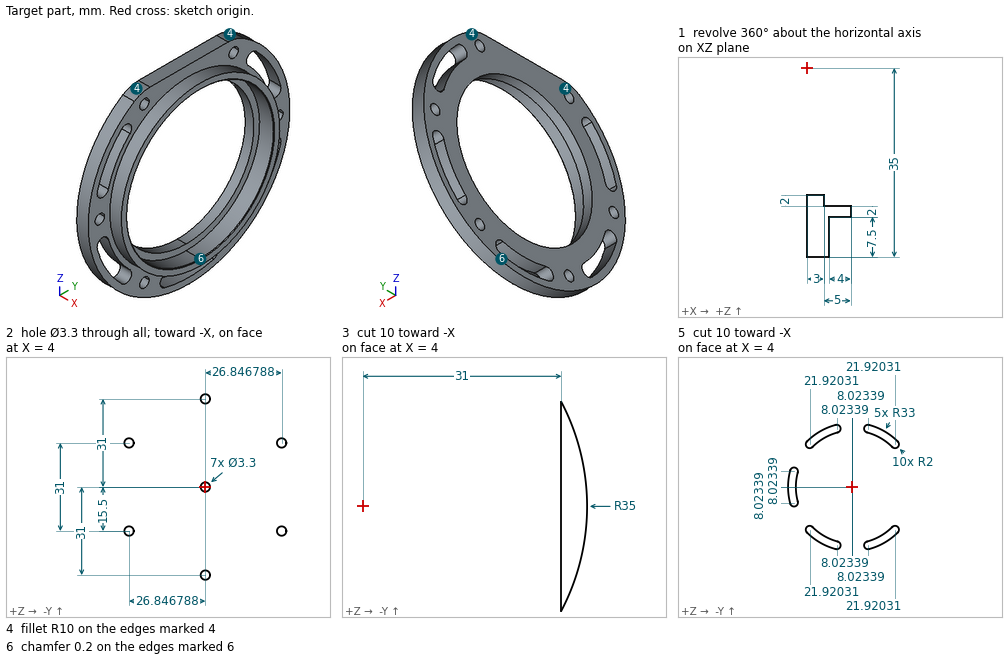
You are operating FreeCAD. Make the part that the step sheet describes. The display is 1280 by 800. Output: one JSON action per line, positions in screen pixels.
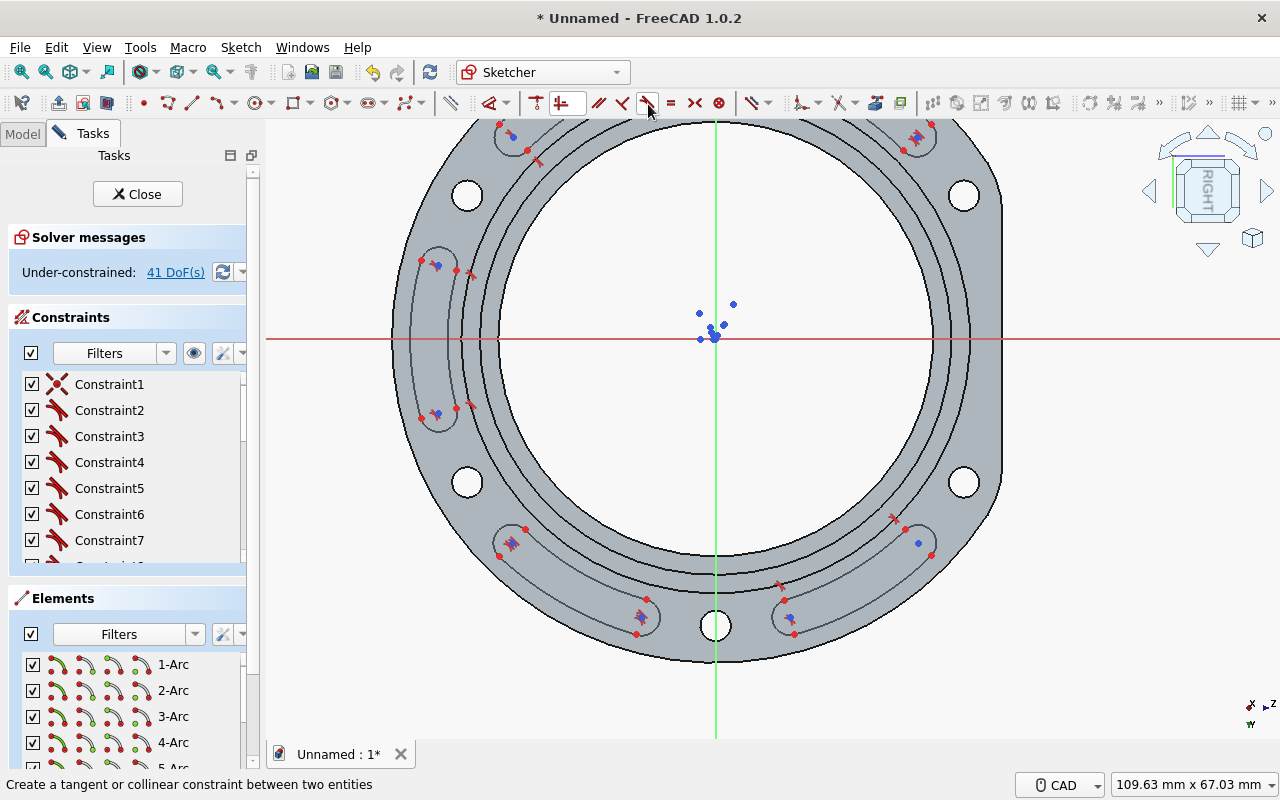
{"action": "left_click", "coordinate": [840, 618]}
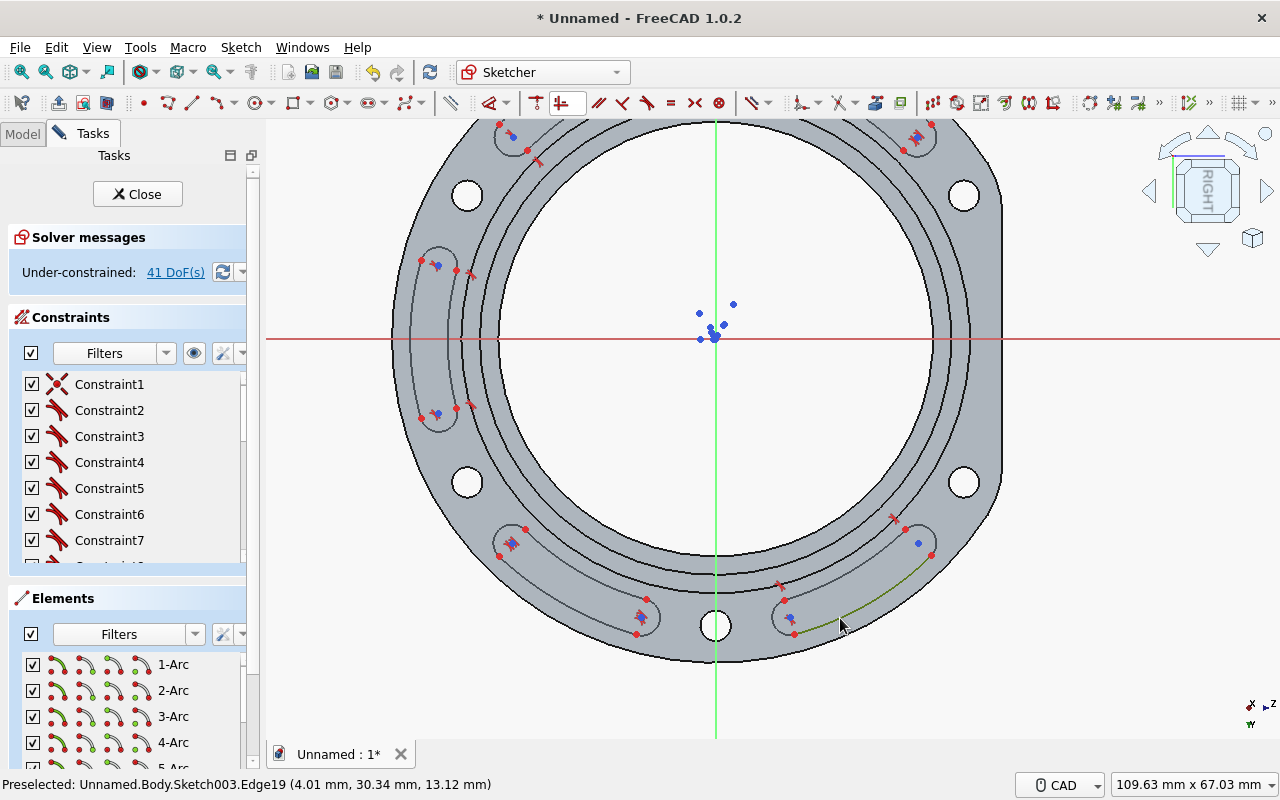
{"action": "left_click", "coordinate": [936, 540]}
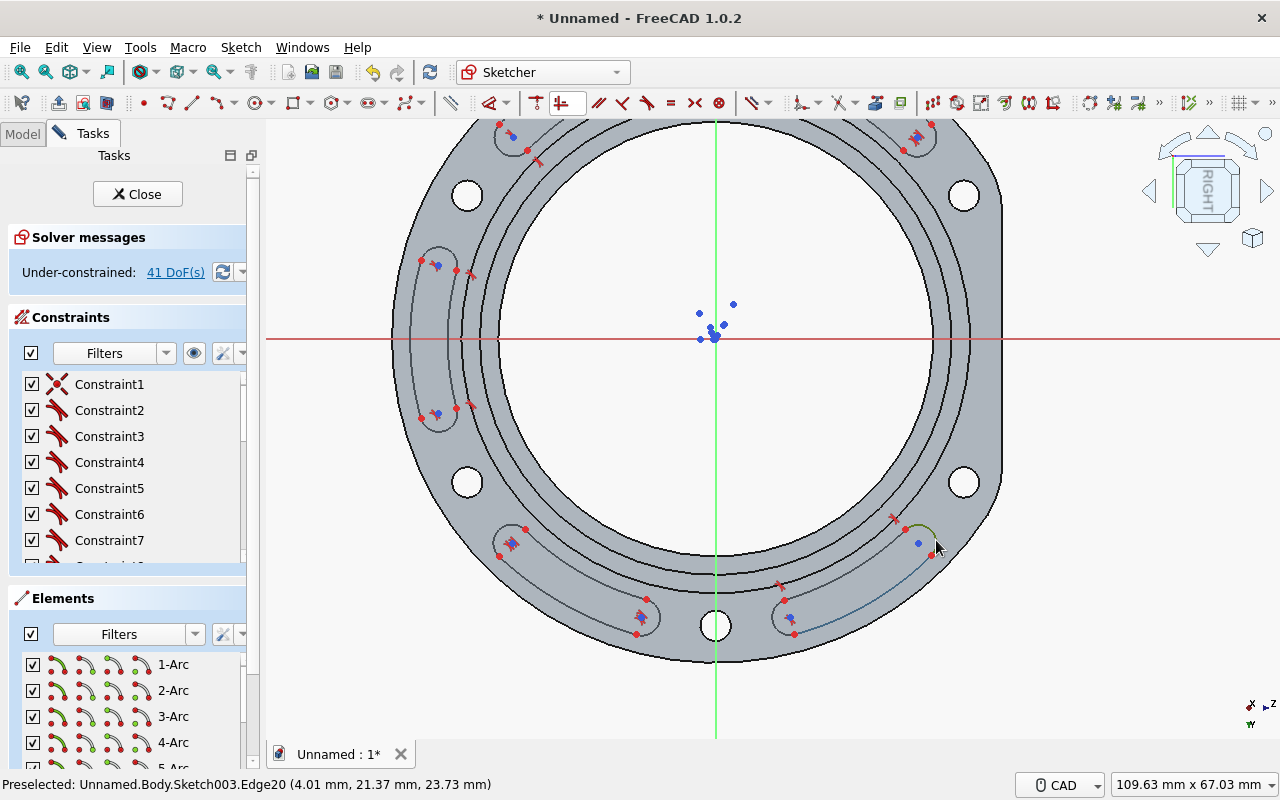
{"action": "left_click", "coordinate": [648, 104]}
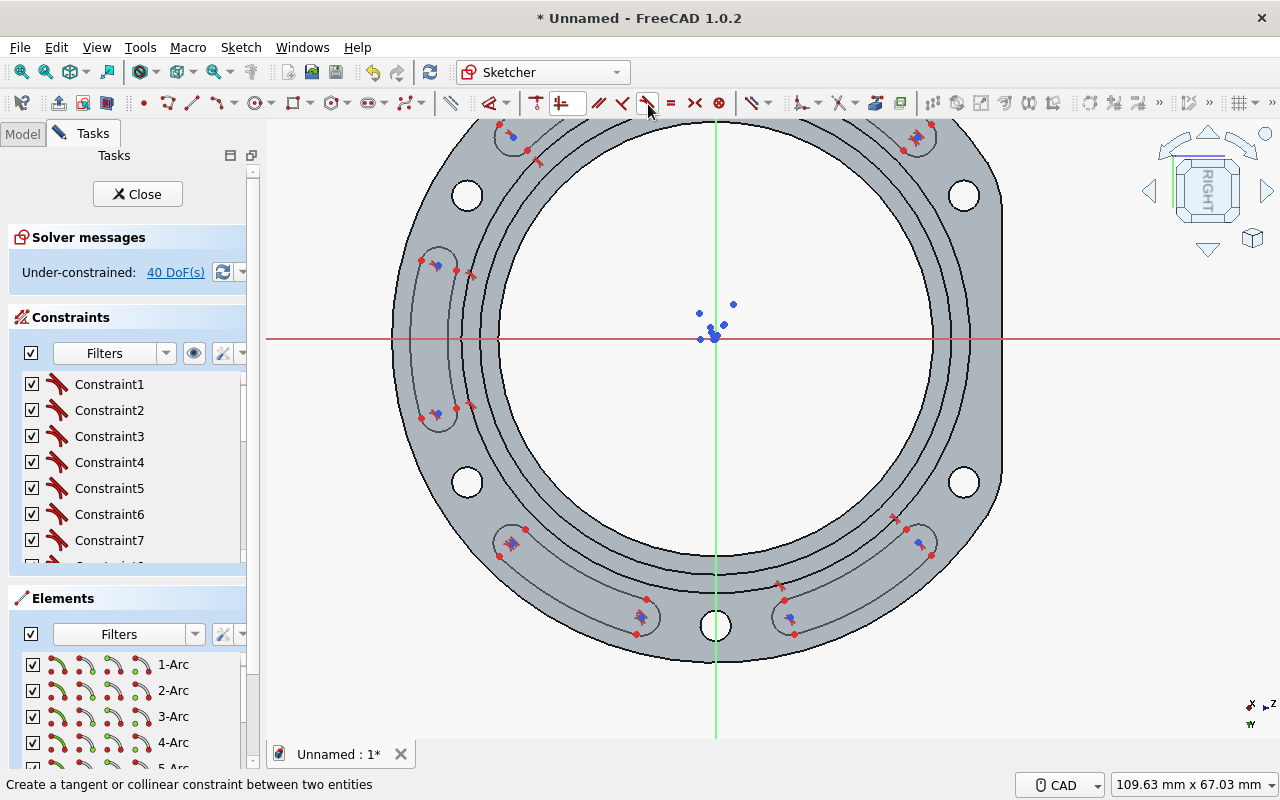
{"action": "left_click", "coordinate": [536, 587]}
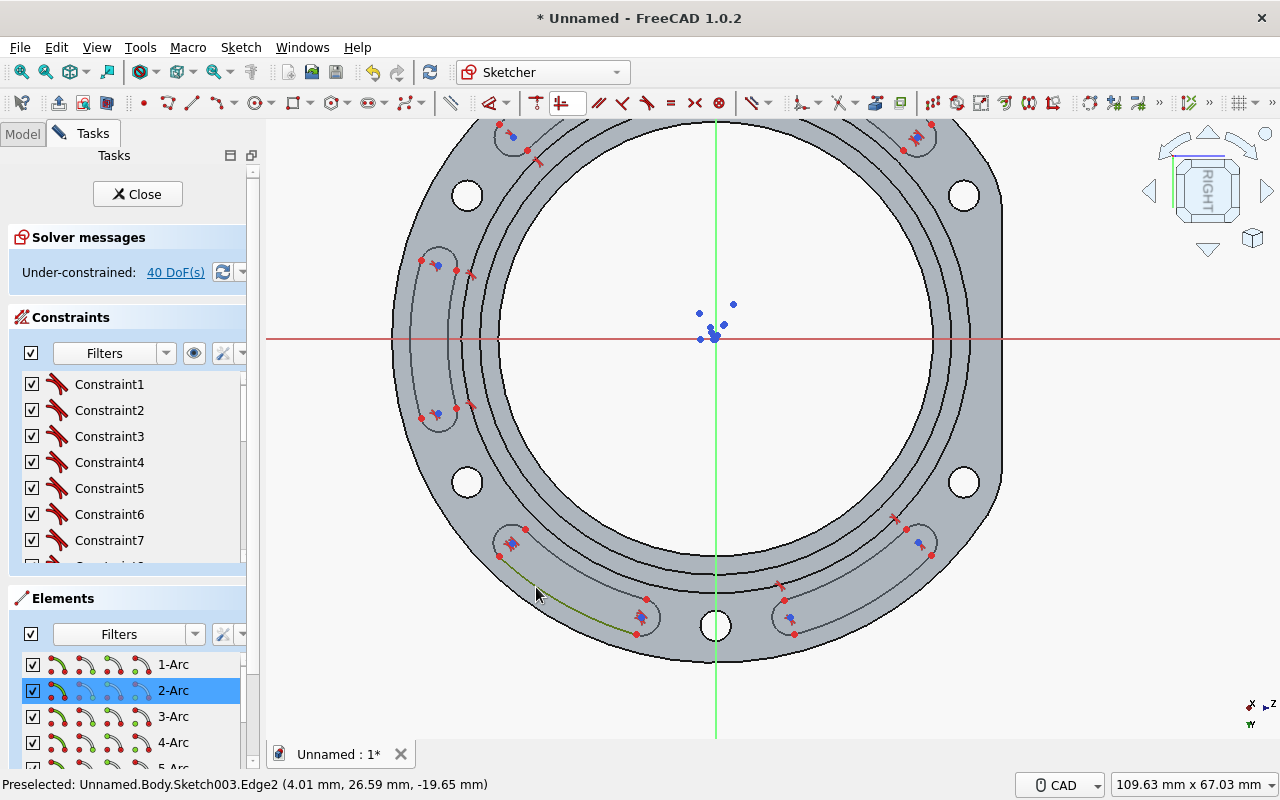
{"action": "left_click", "coordinate": [557, 557]}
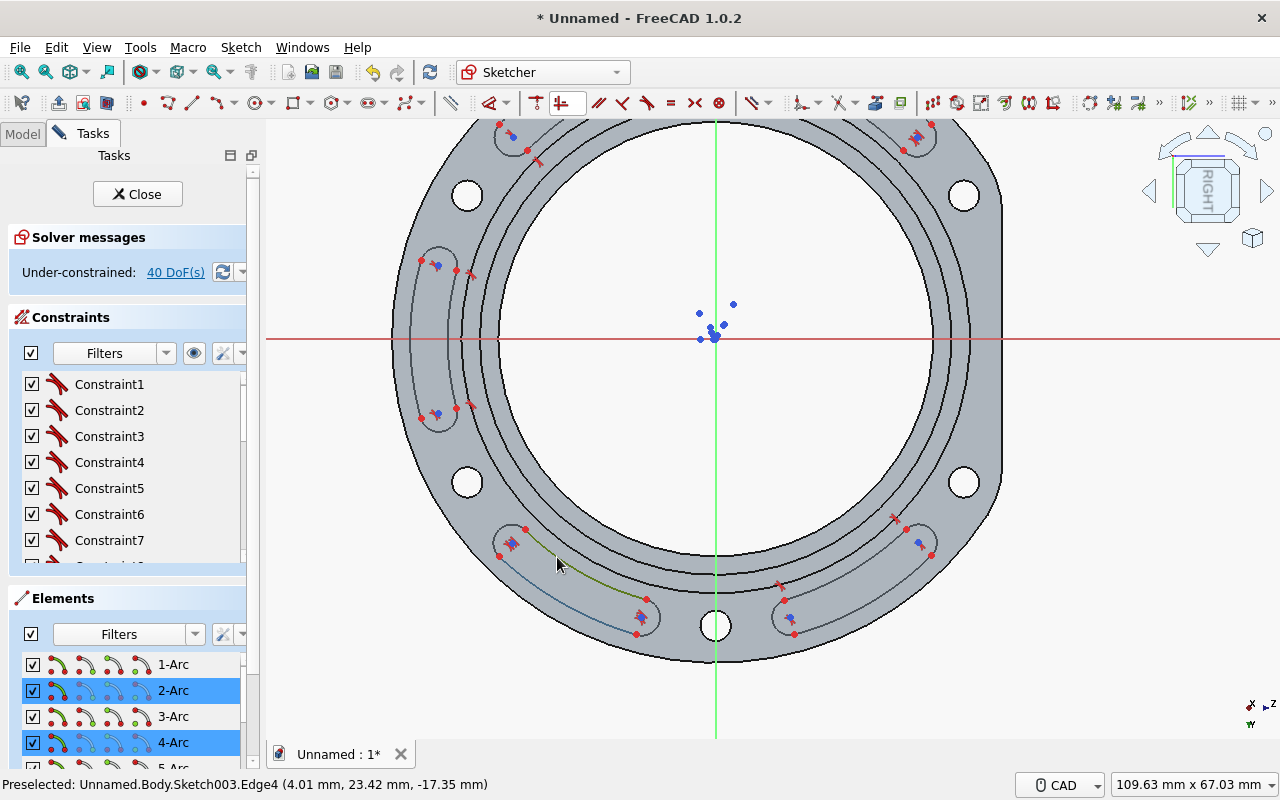
{"action": "left_click", "coordinate": [536, 104]}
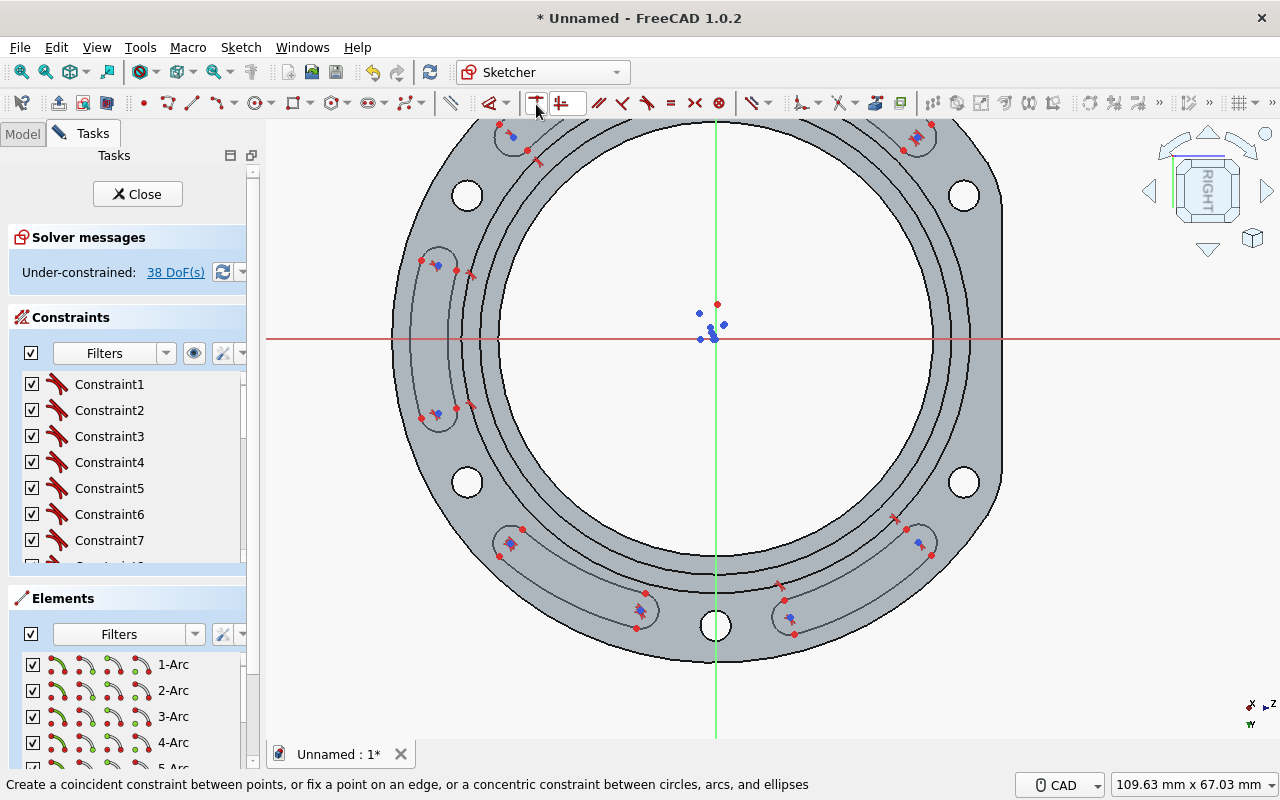
{"action": "left_click", "coordinate": [537, 585]}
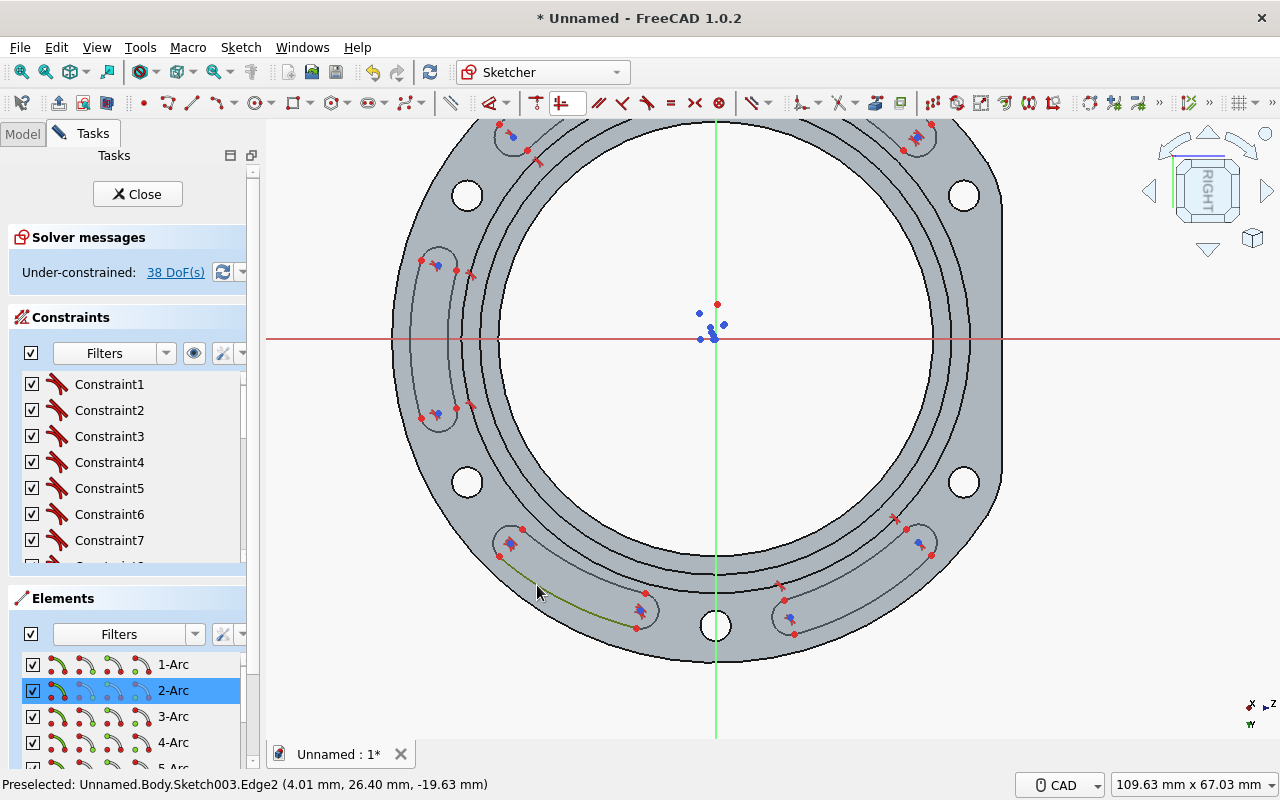
{"action": "left_click", "coordinate": [449, 312]}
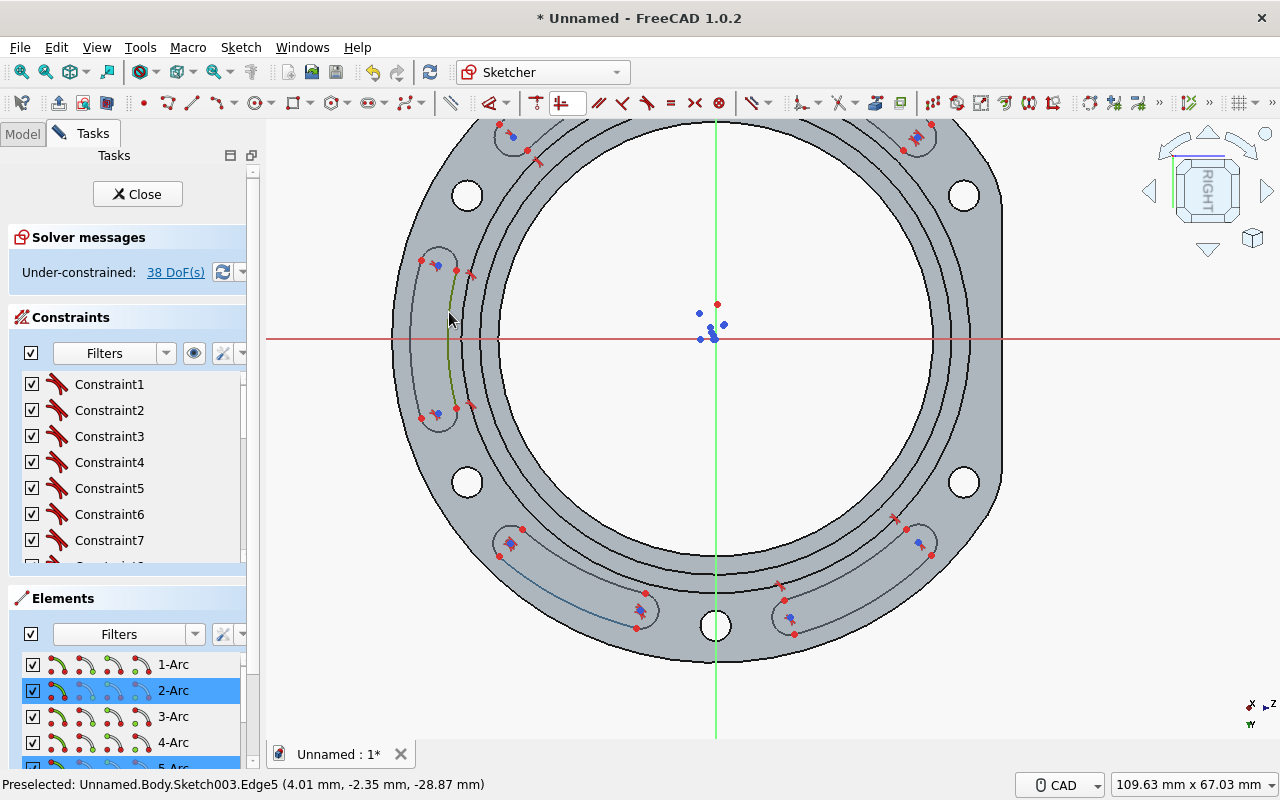
{"action": "left_click", "coordinate": [536, 104]}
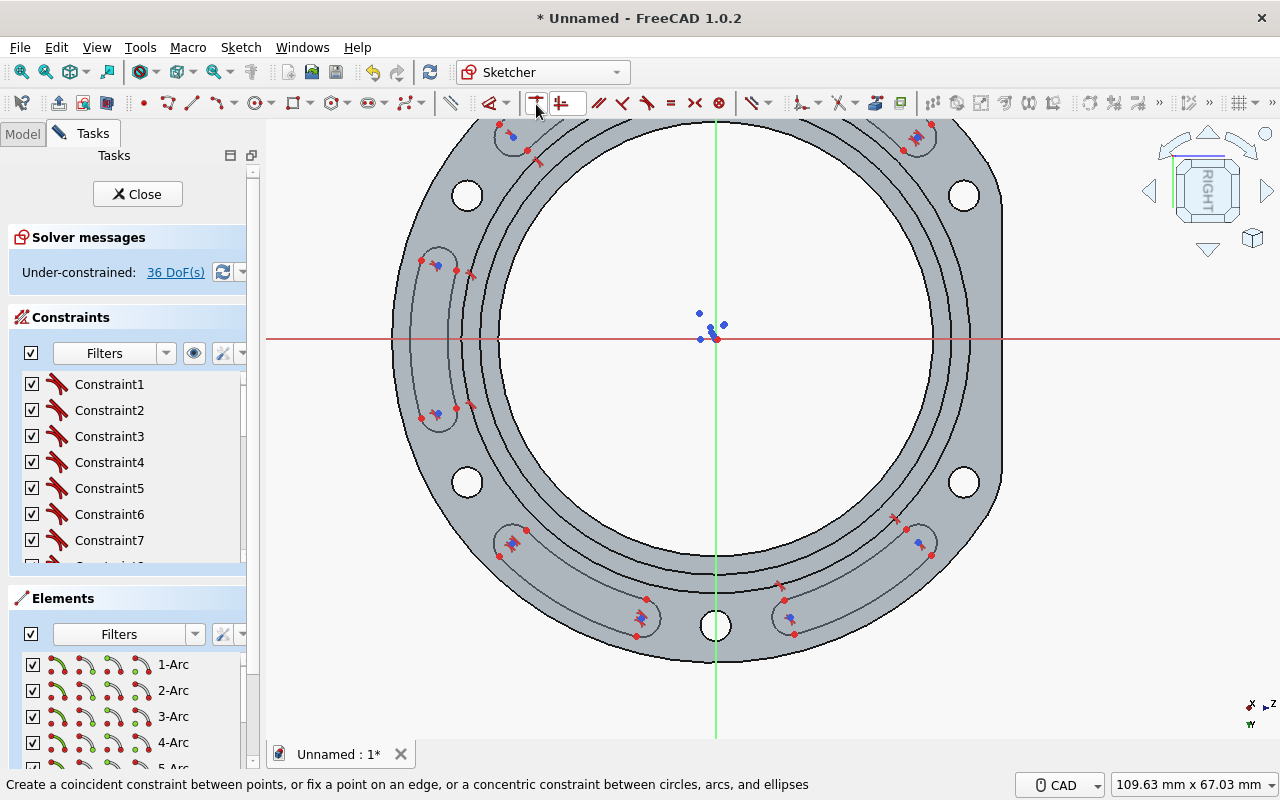
{"action": "left_click", "coordinate": [536, 588]}